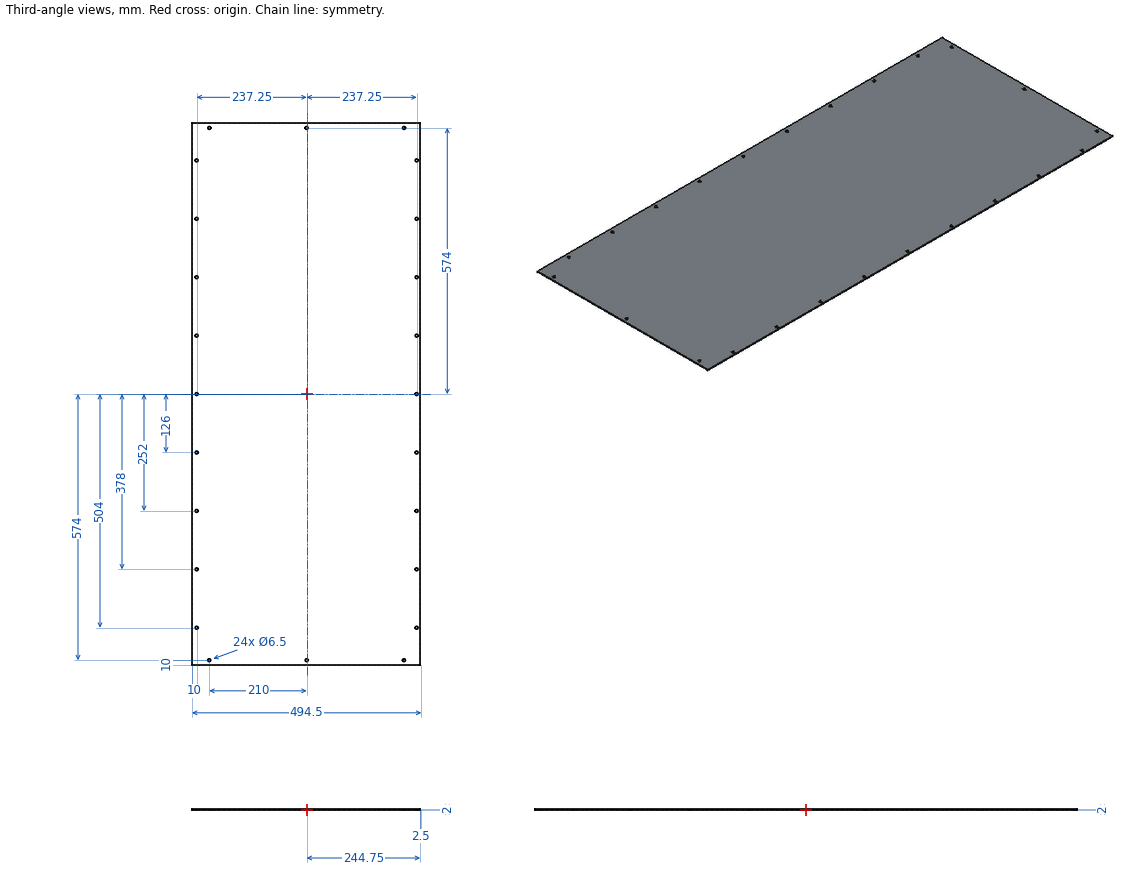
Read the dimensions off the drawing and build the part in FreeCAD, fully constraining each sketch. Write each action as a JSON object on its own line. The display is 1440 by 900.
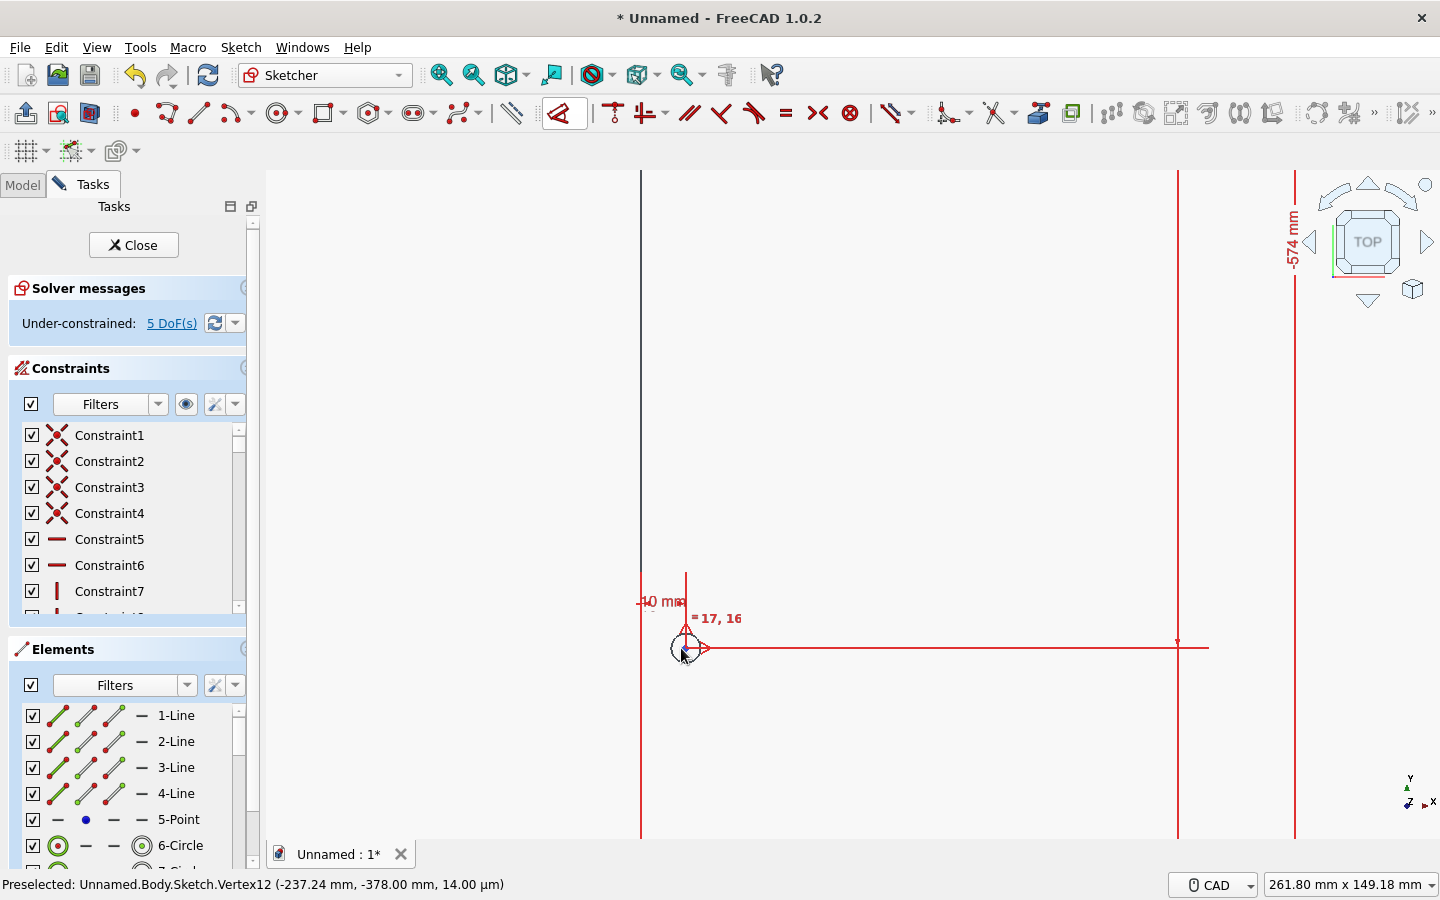
{"action": "scroll", "coordinate": [689, 659], "scroll_direction": "down", "scroll_amount": 12}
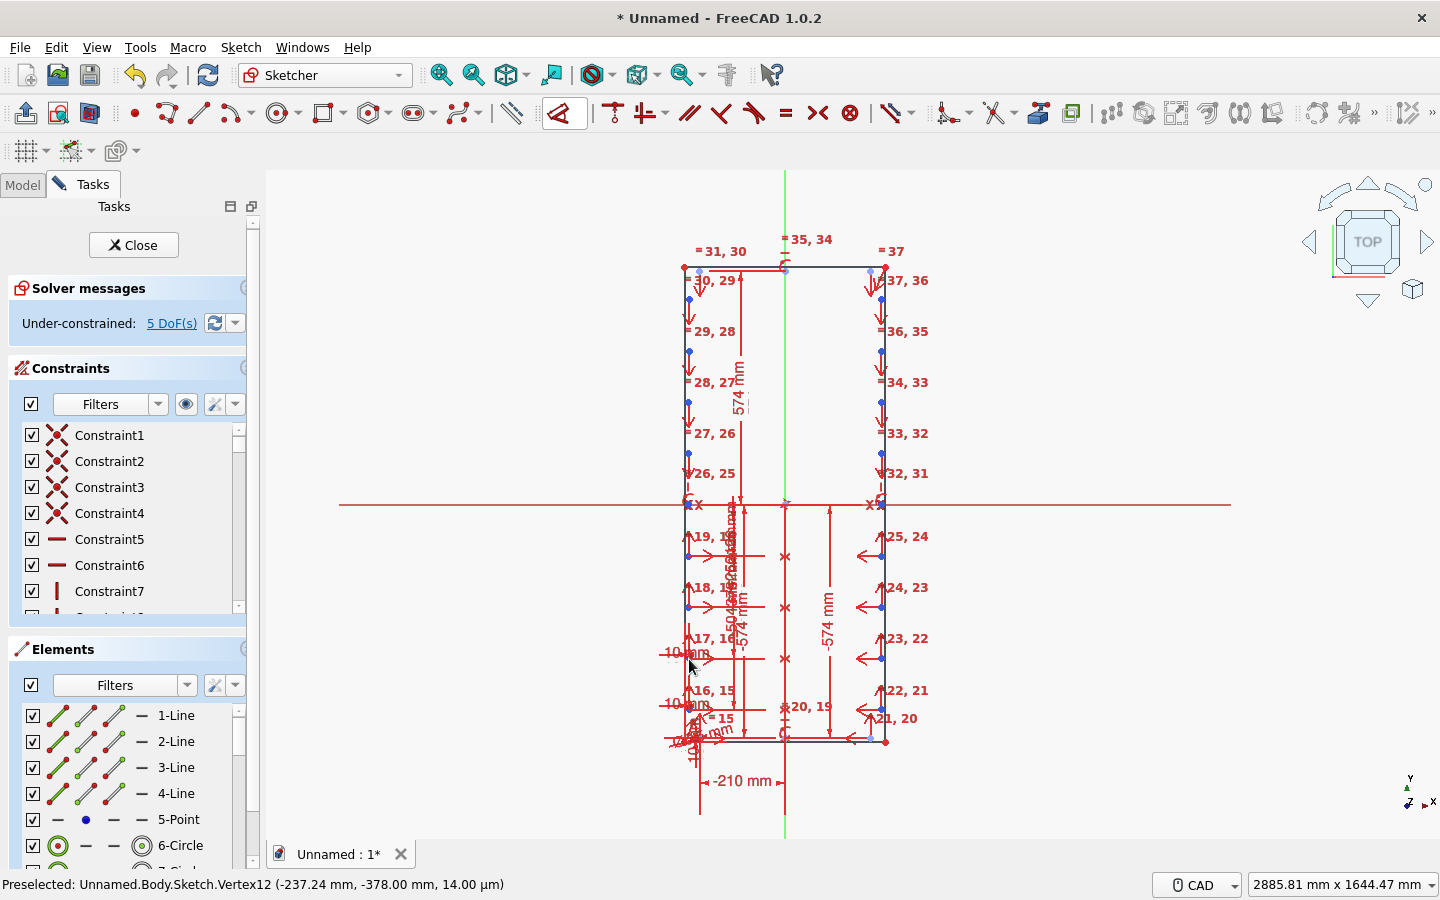
{"action": "scroll", "coordinate": [685, 742], "scroll_direction": "up", "scroll_amount": 12}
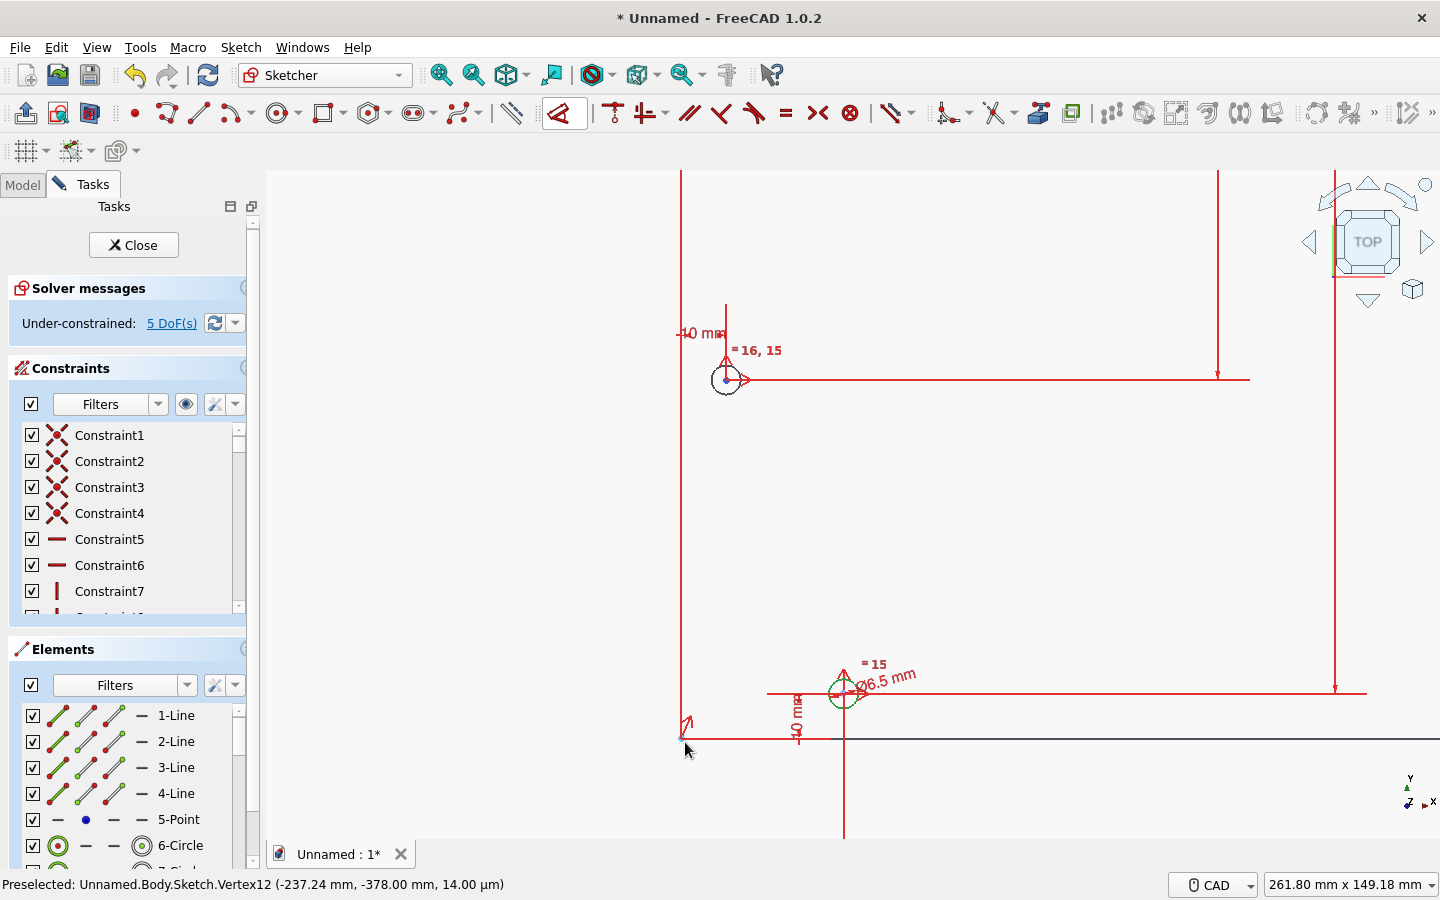
{"action": "left_click", "coordinate": [681, 739]}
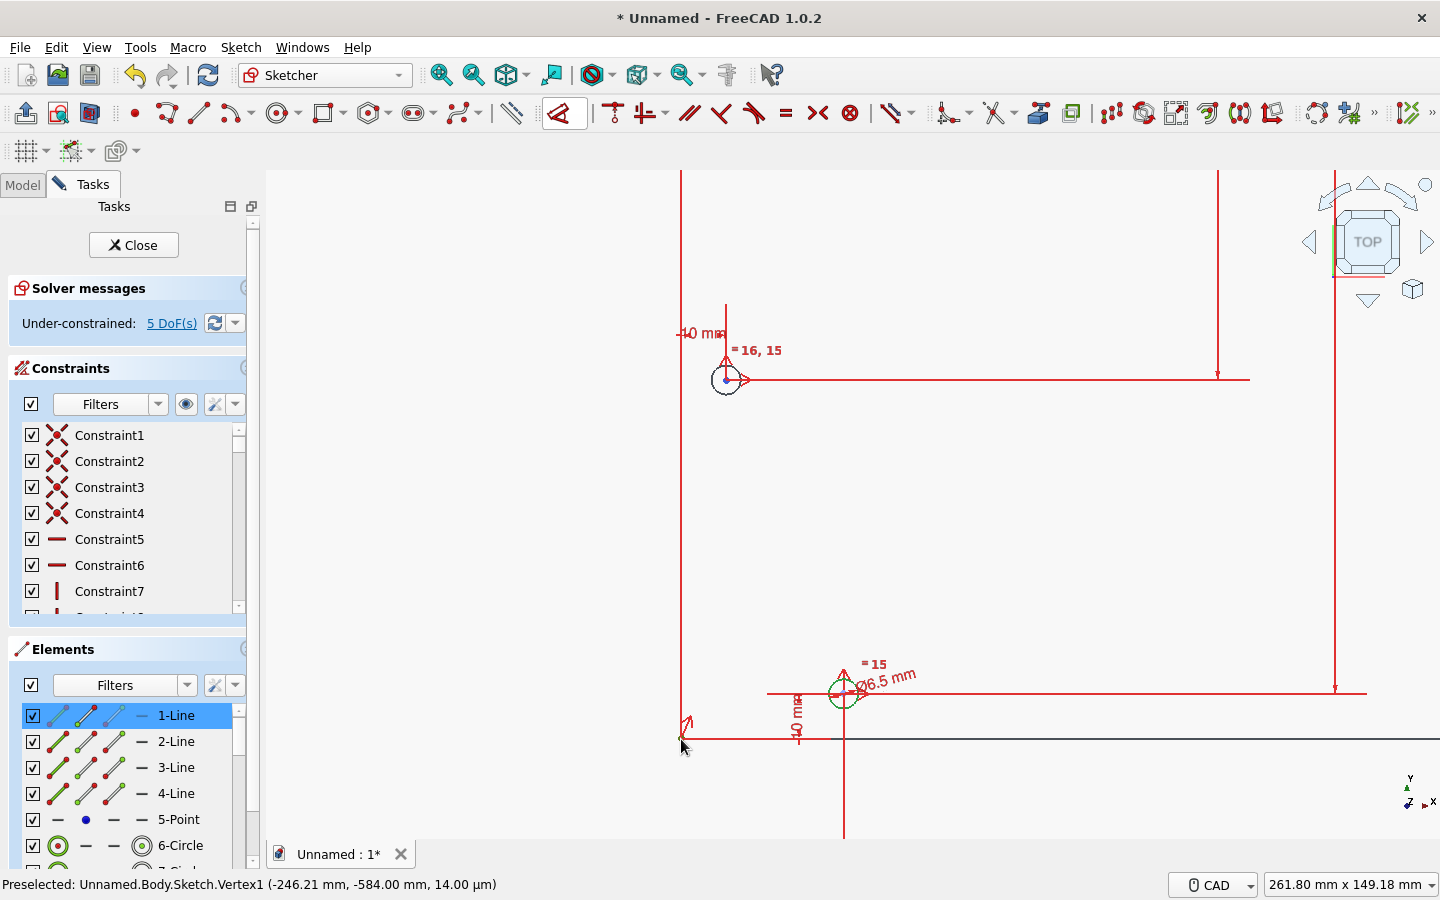
{"action": "scroll", "coordinate": [685, 742], "scroll_direction": "down", "scroll_amount": 12}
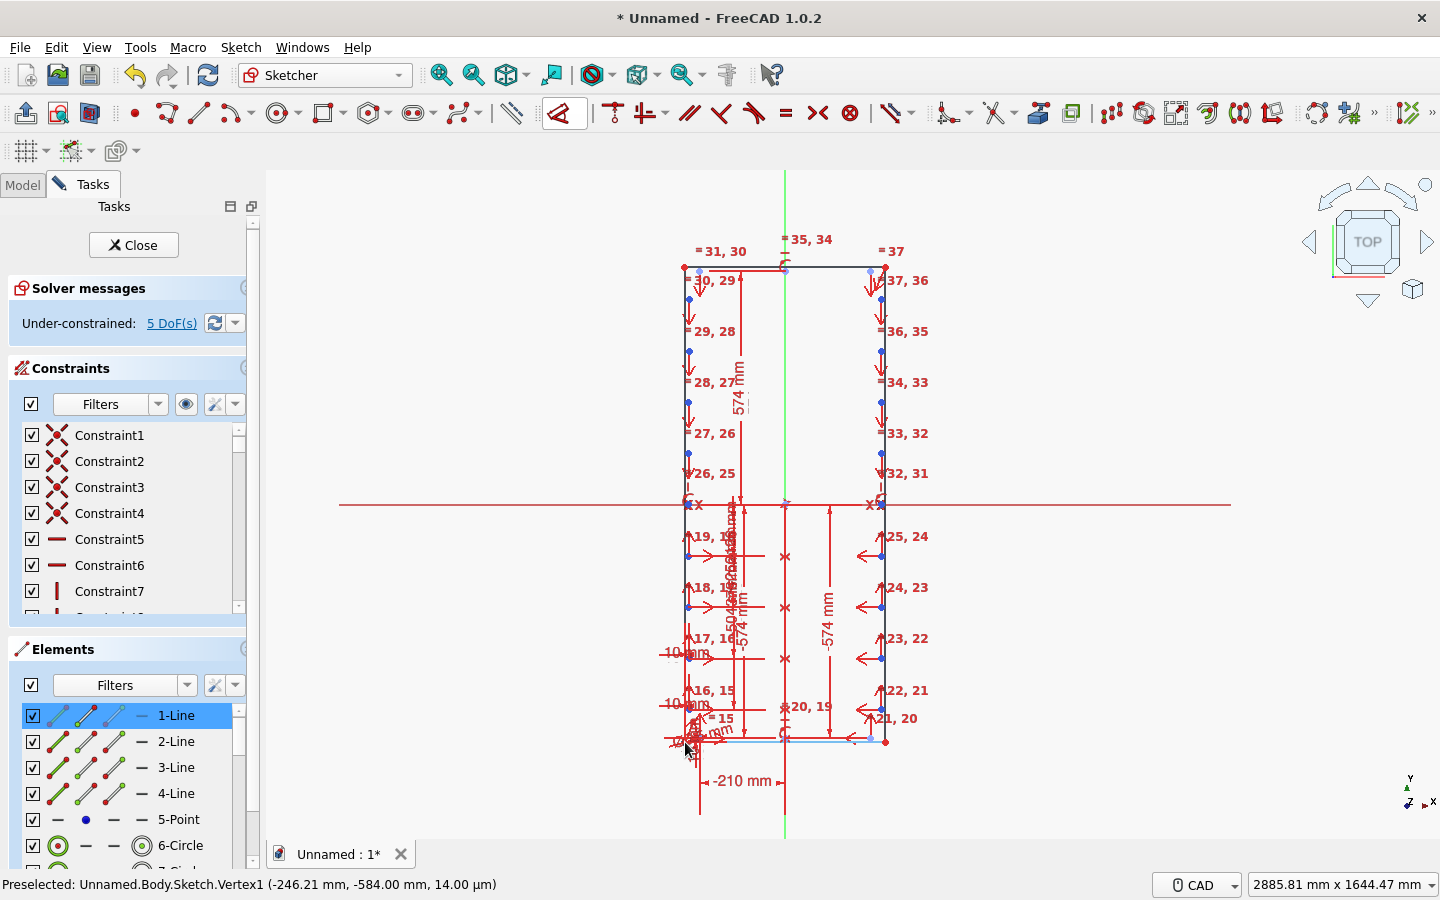
{"action": "scroll", "coordinate": [689, 607], "scroll_direction": "up", "scroll_amount": 12}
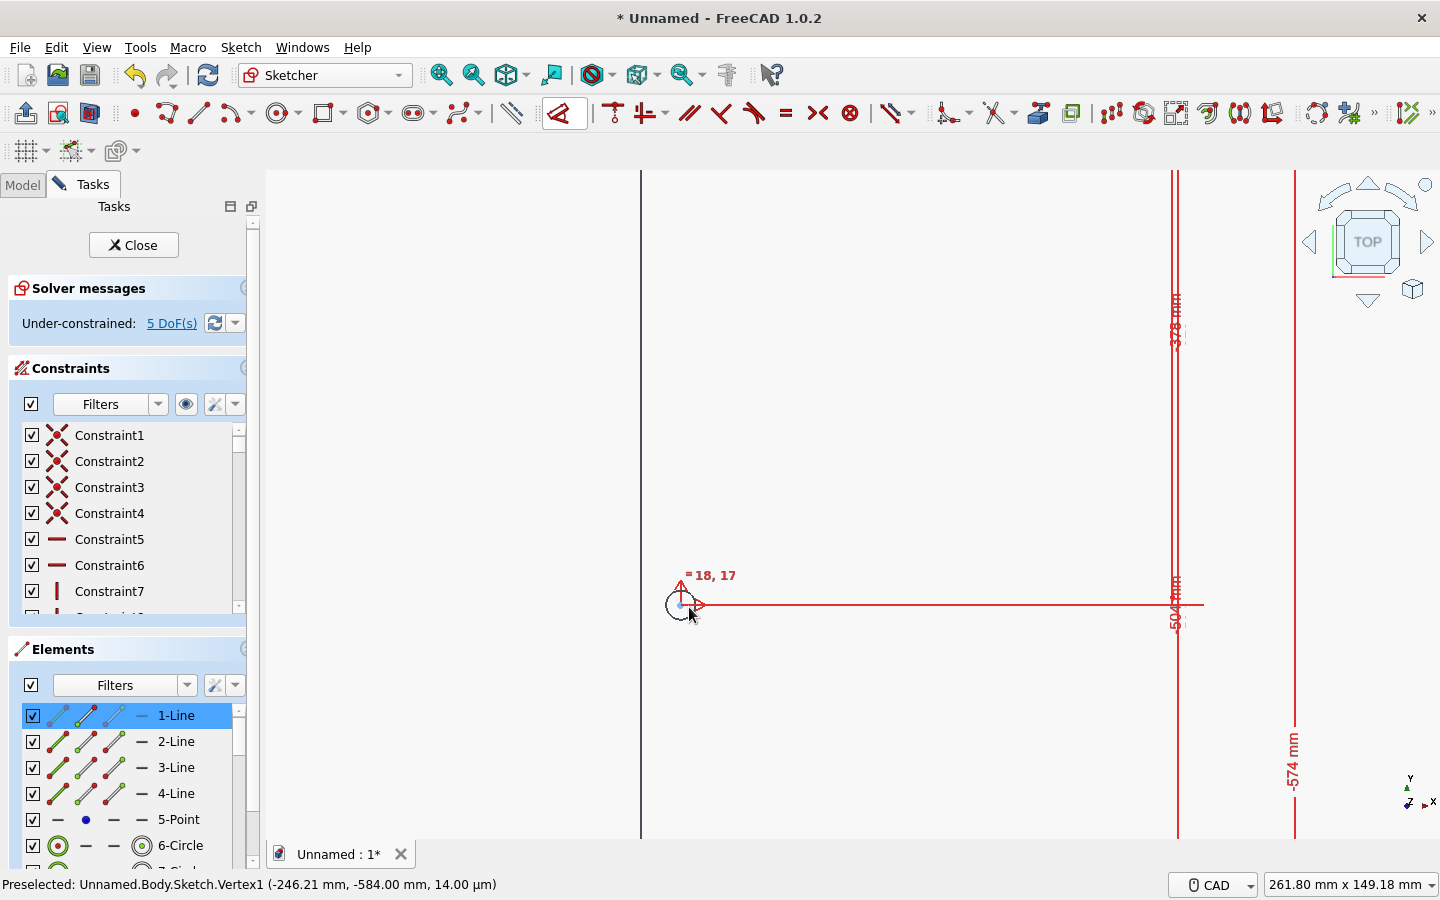
{"action": "left_click", "coordinate": [681, 605]}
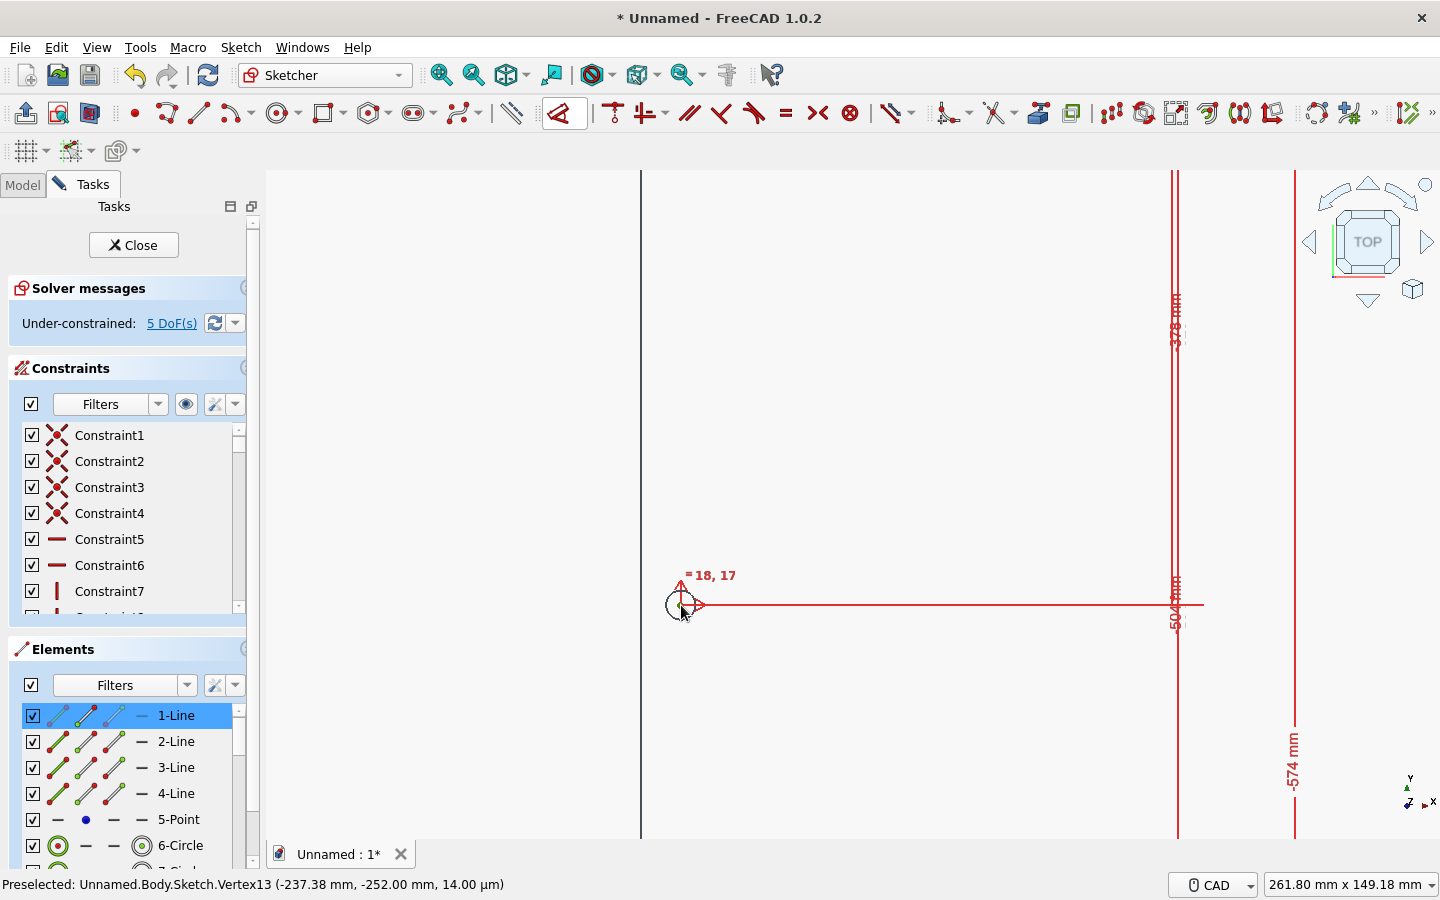
{"action": "key", "text": "l"}